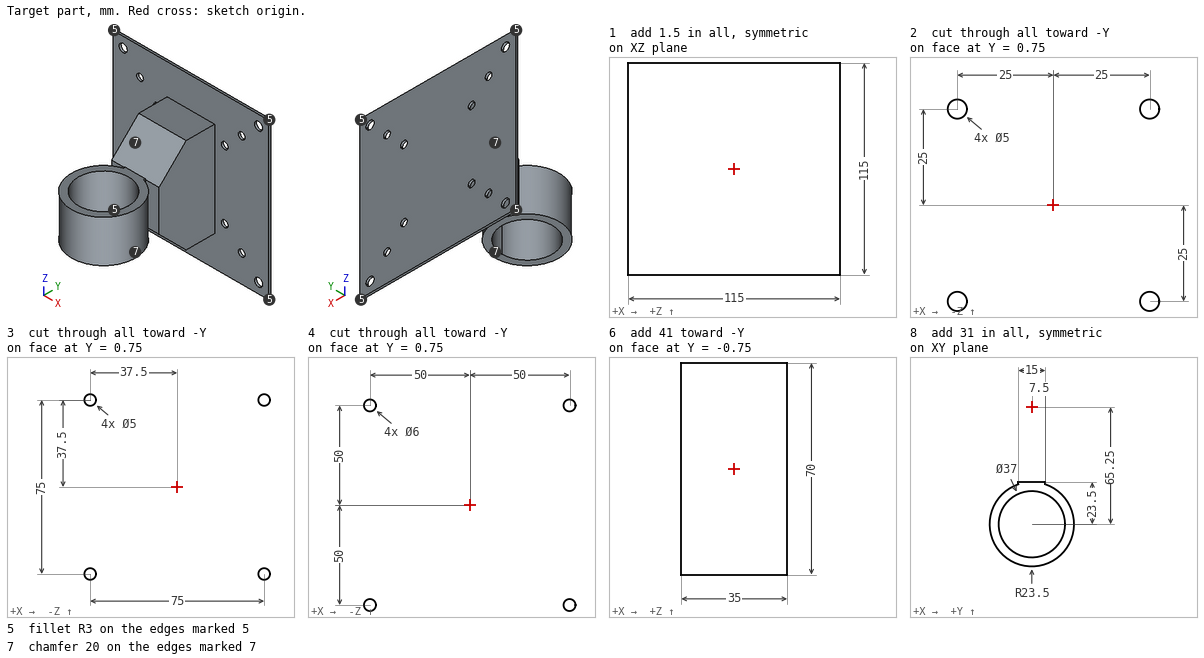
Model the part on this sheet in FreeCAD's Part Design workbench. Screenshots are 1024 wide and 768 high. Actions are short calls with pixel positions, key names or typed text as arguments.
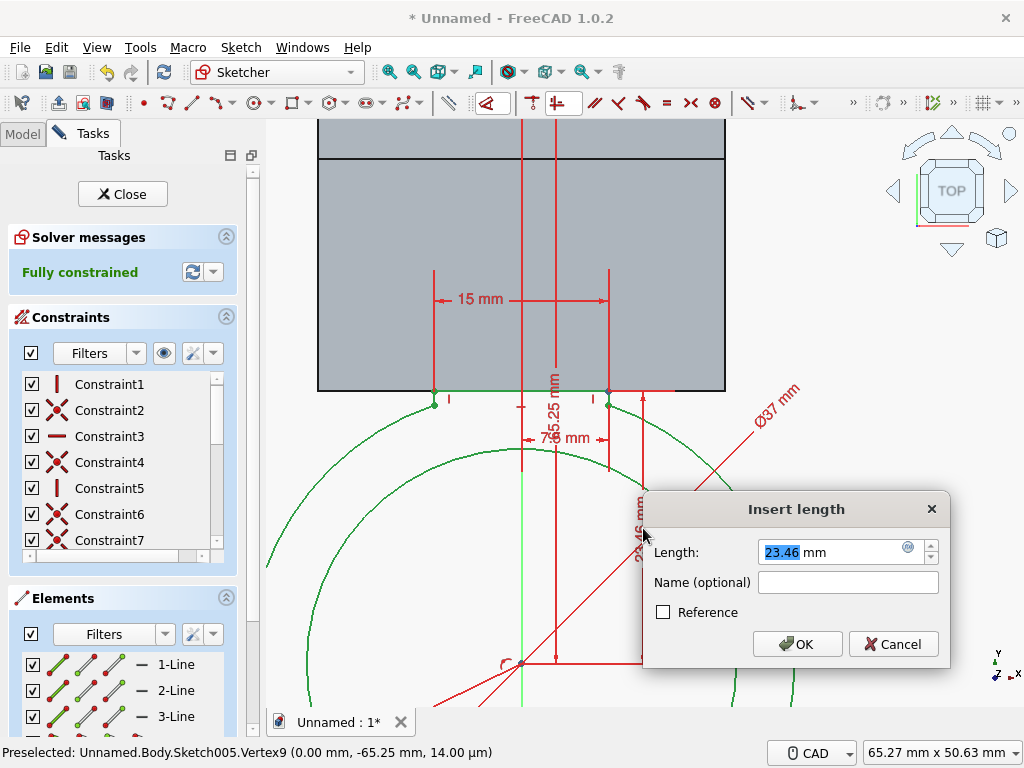
text(23.5)
key(Return)
key(Escape)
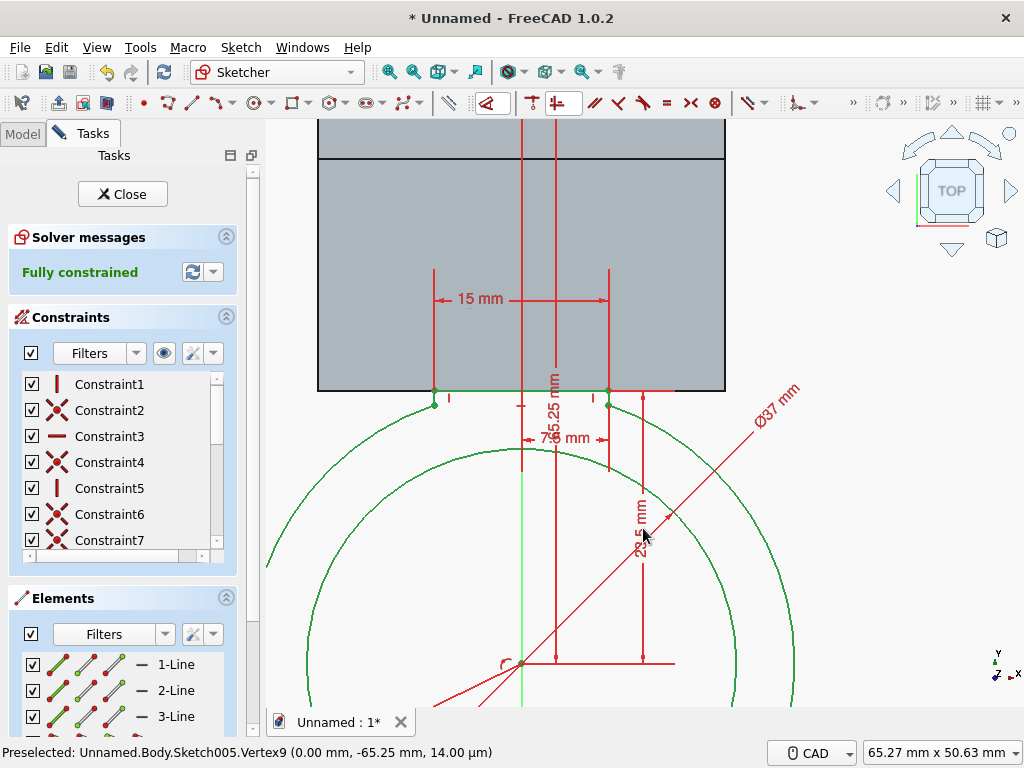
click(123, 194)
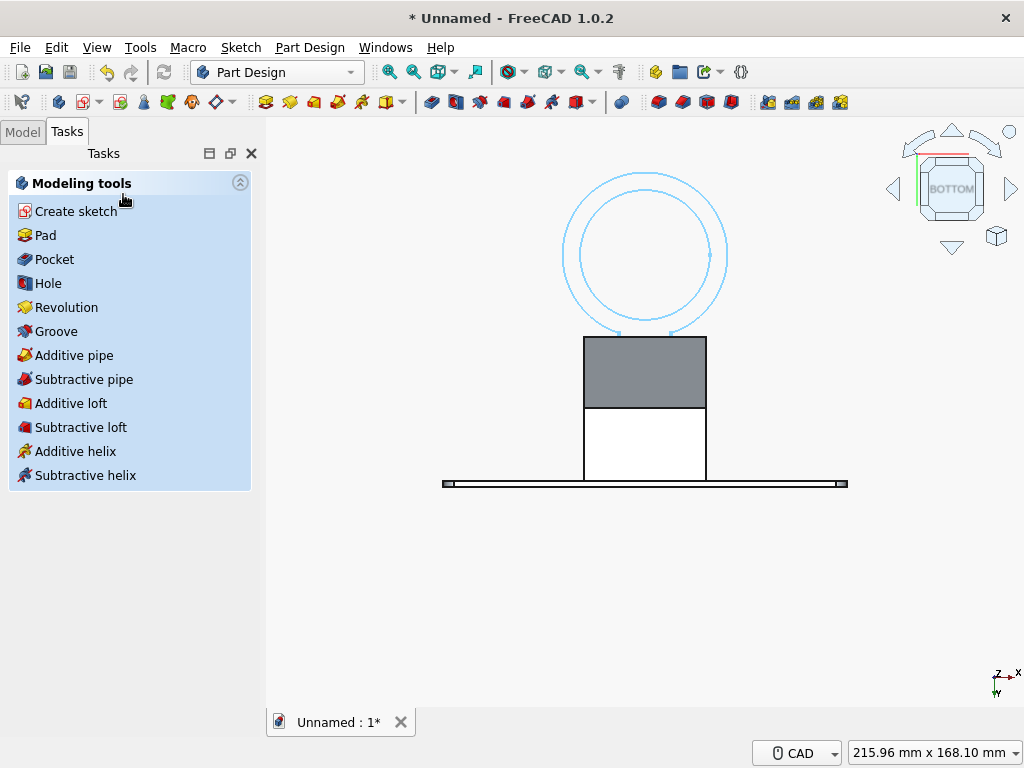
click(266, 102)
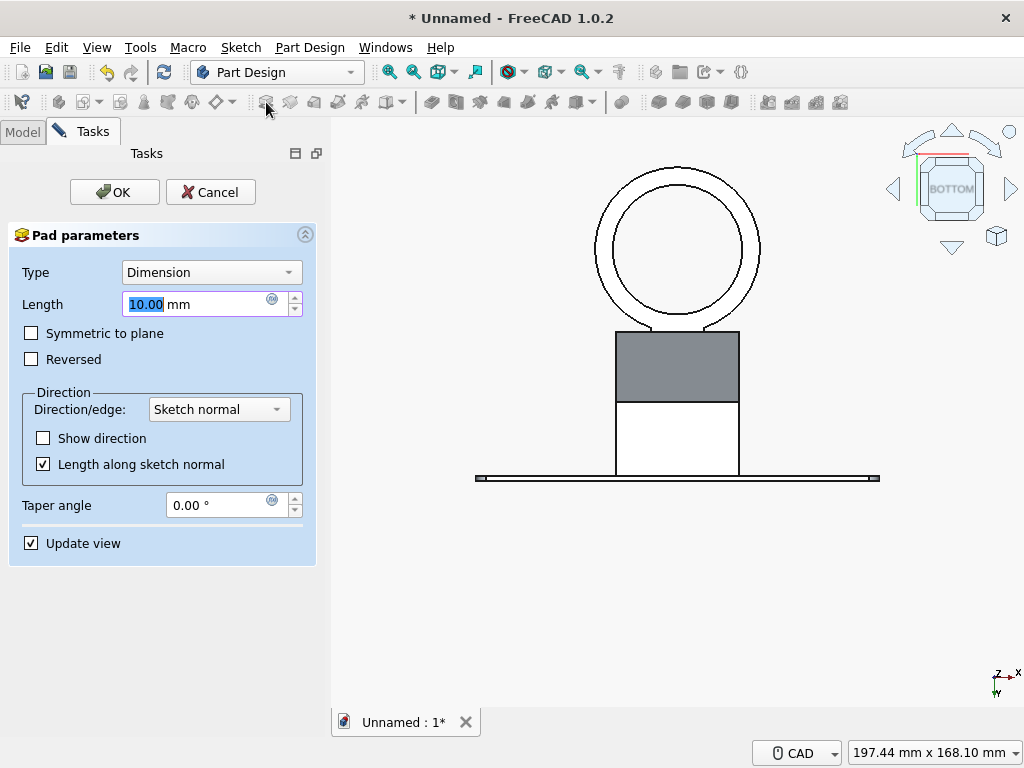
text(31)
key(Tab)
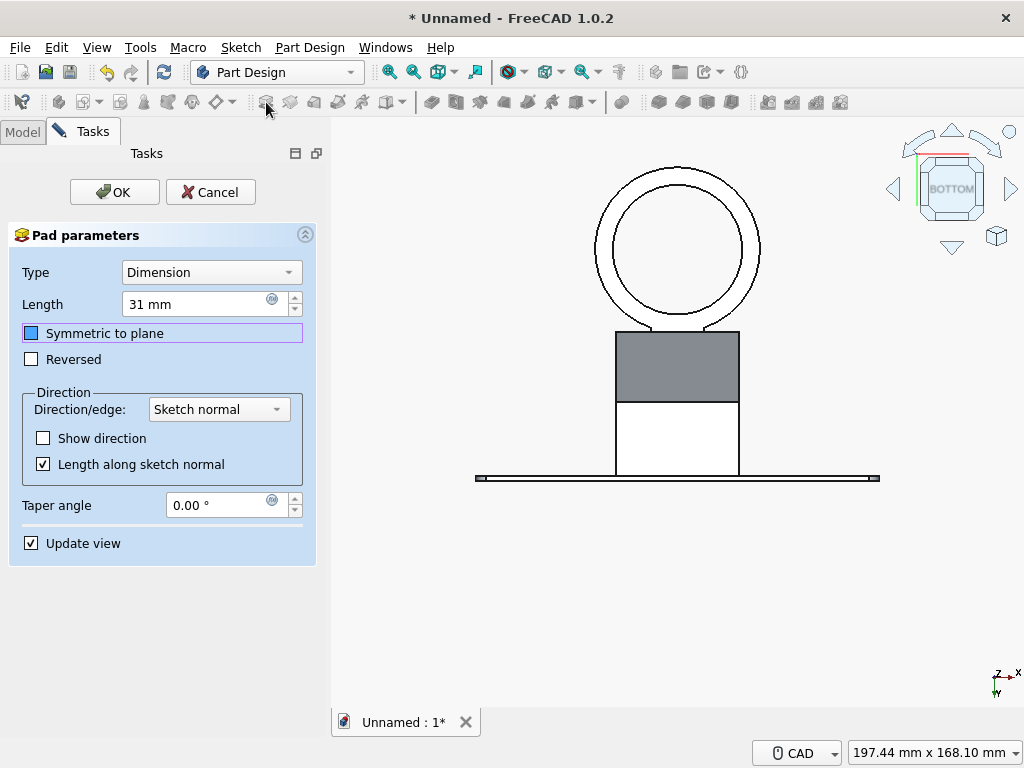
click(30, 333)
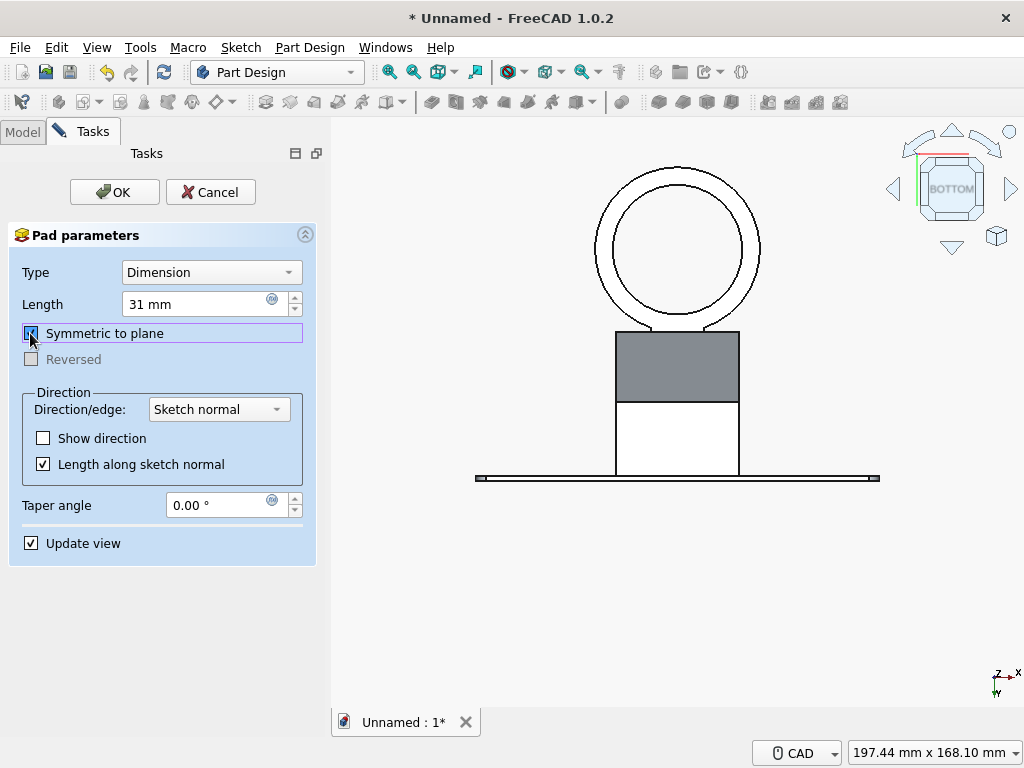
click(115, 192)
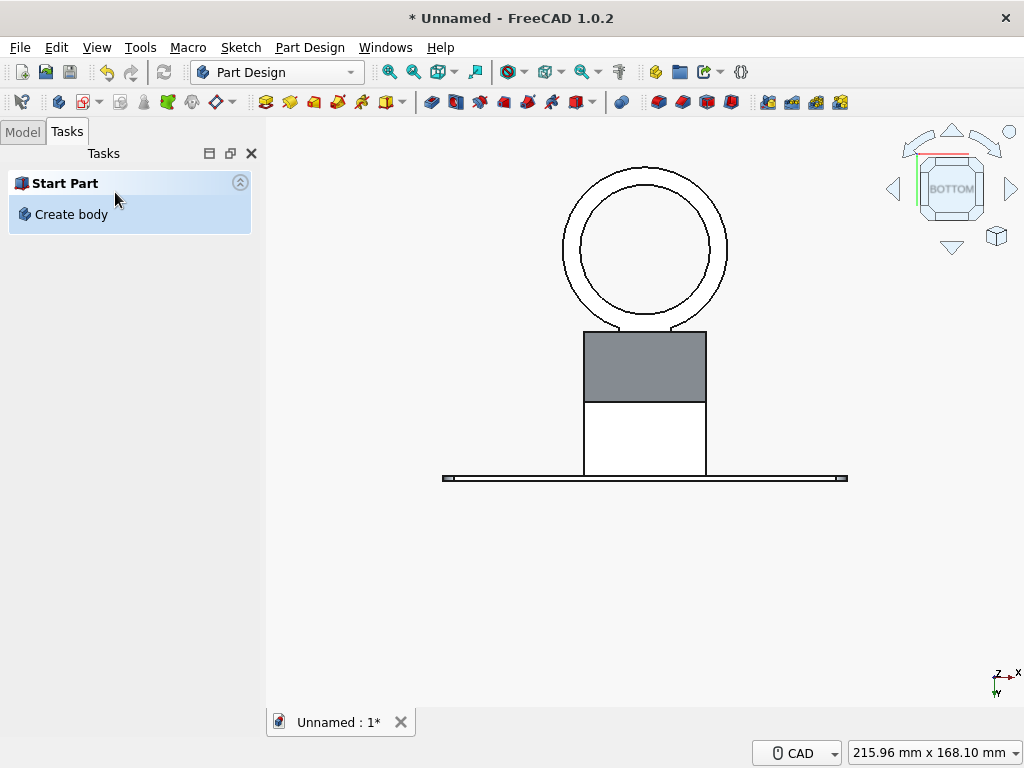
key(0)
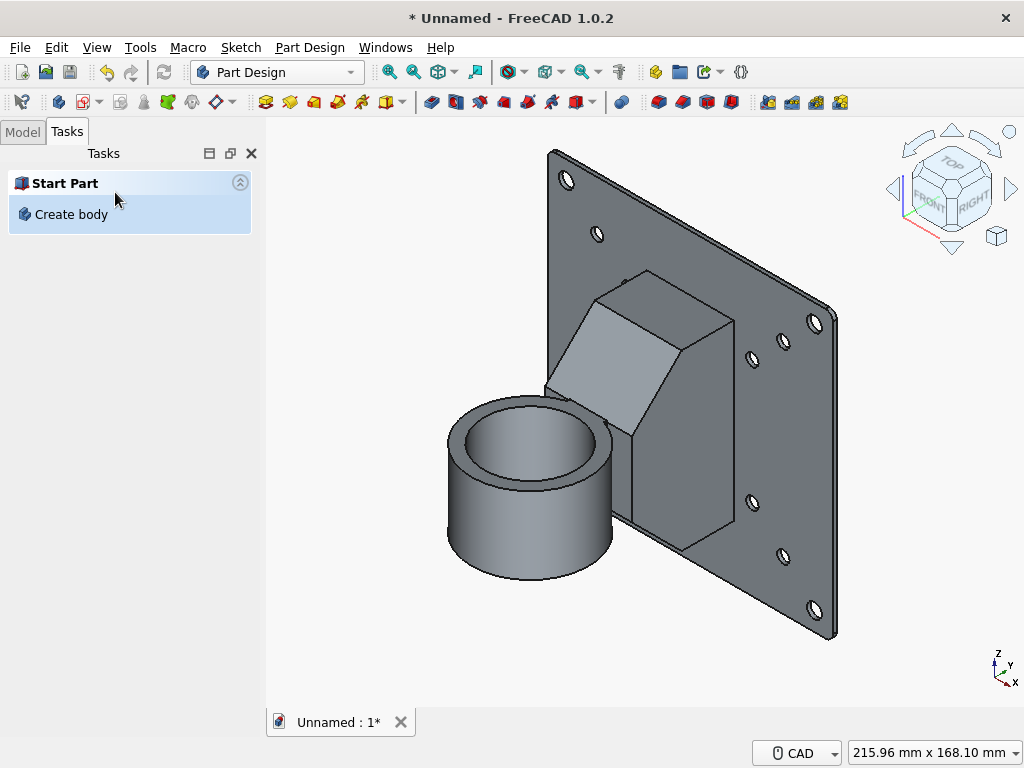
click(390, 72)